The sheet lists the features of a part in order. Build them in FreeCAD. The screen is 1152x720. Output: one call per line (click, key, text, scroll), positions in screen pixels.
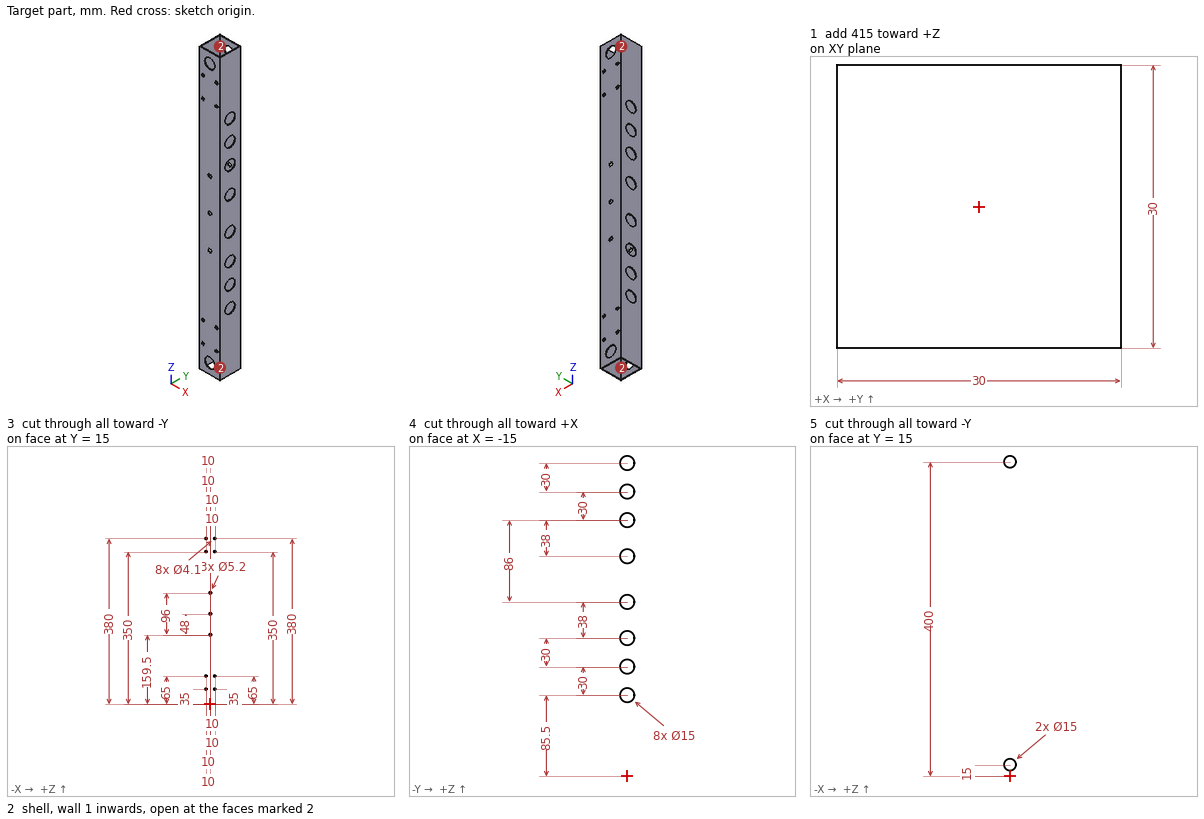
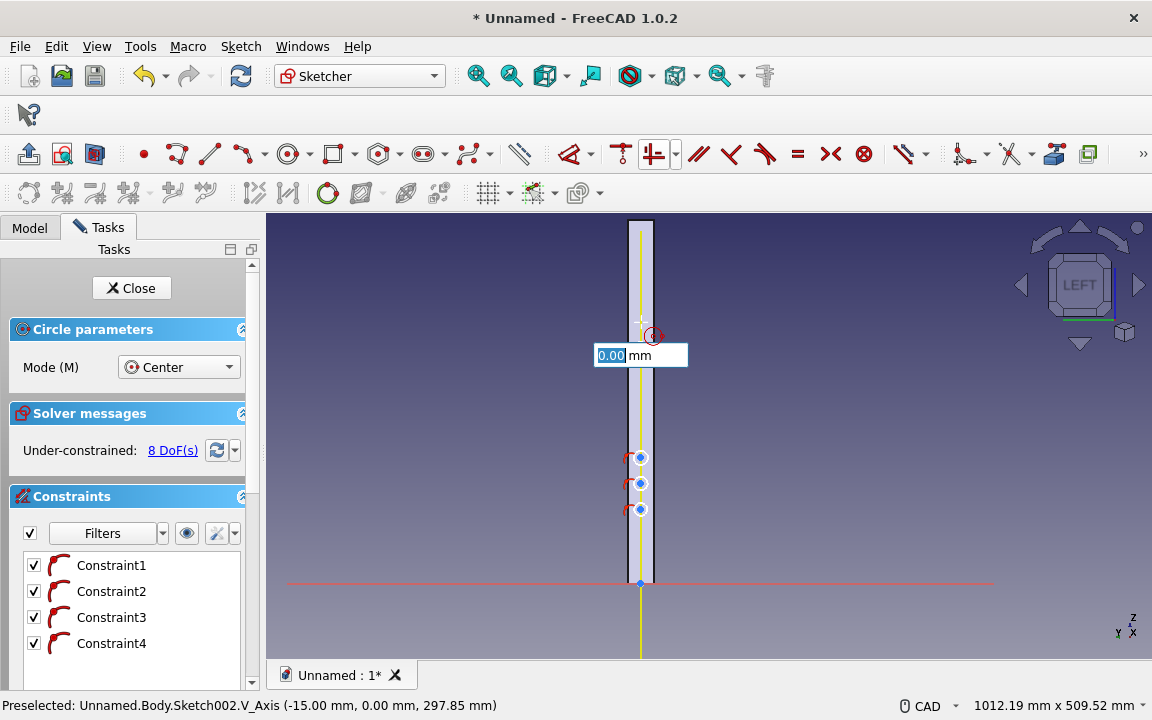
scroll(647, 319, up, 5)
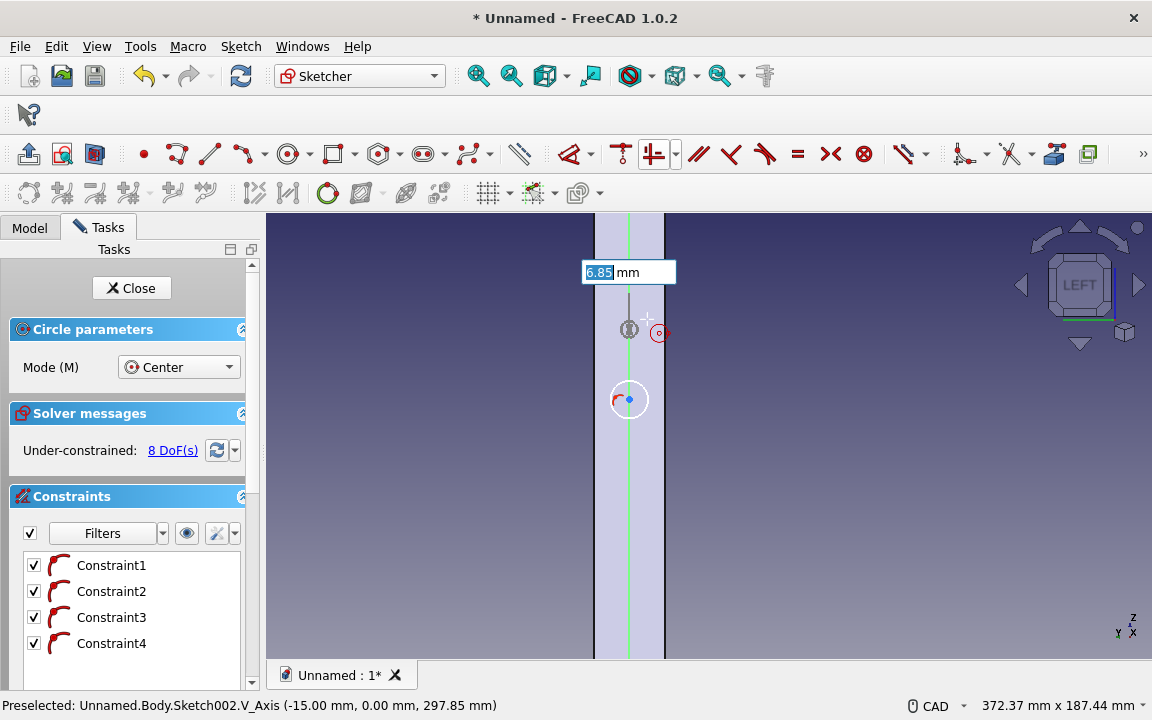
click(646, 319)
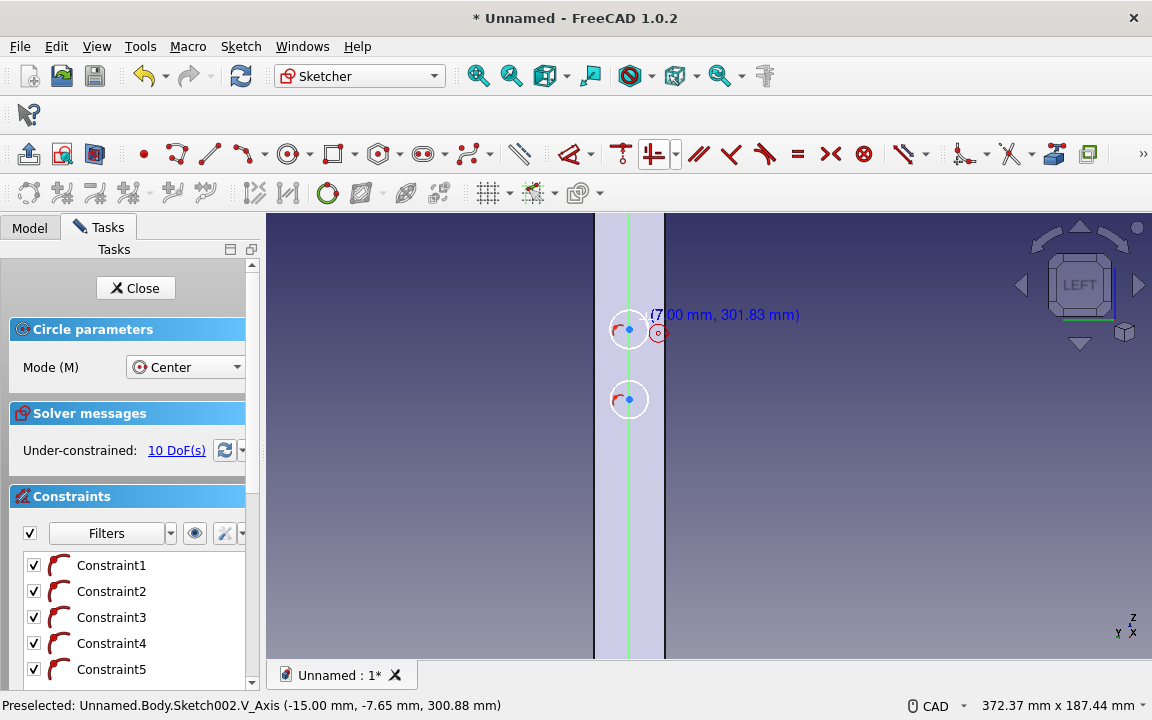
scroll(629, 254, up, 2)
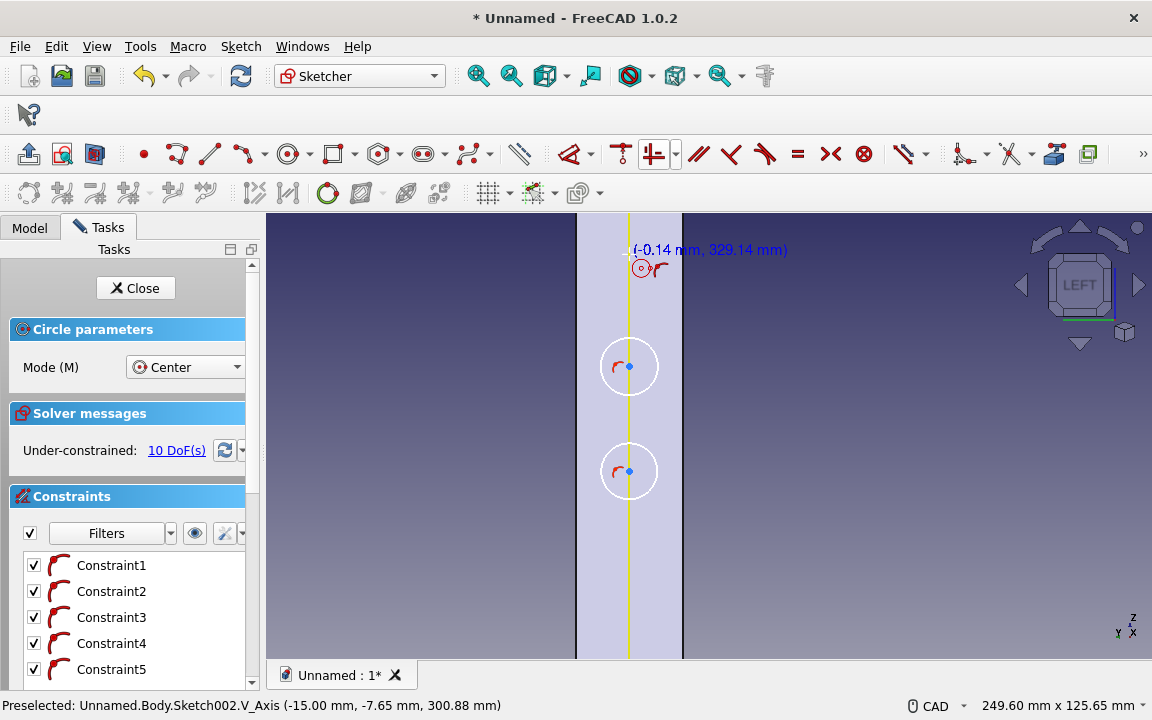
scroll(644, 308, down, 7)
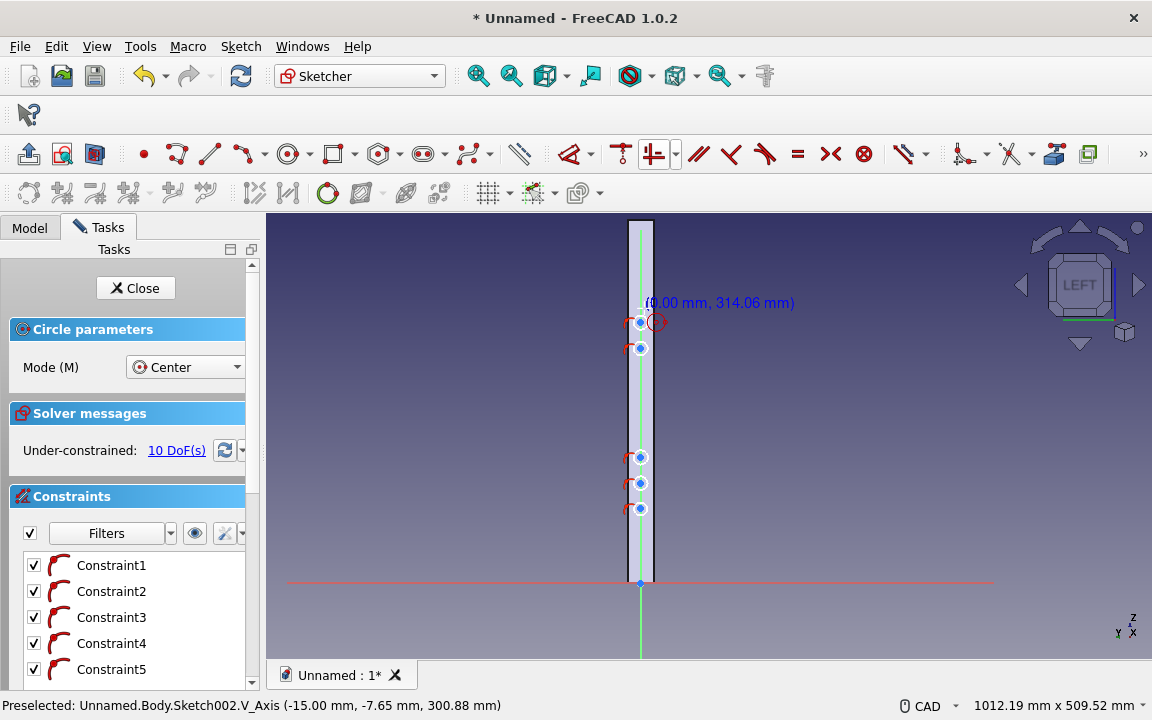
click(641, 295)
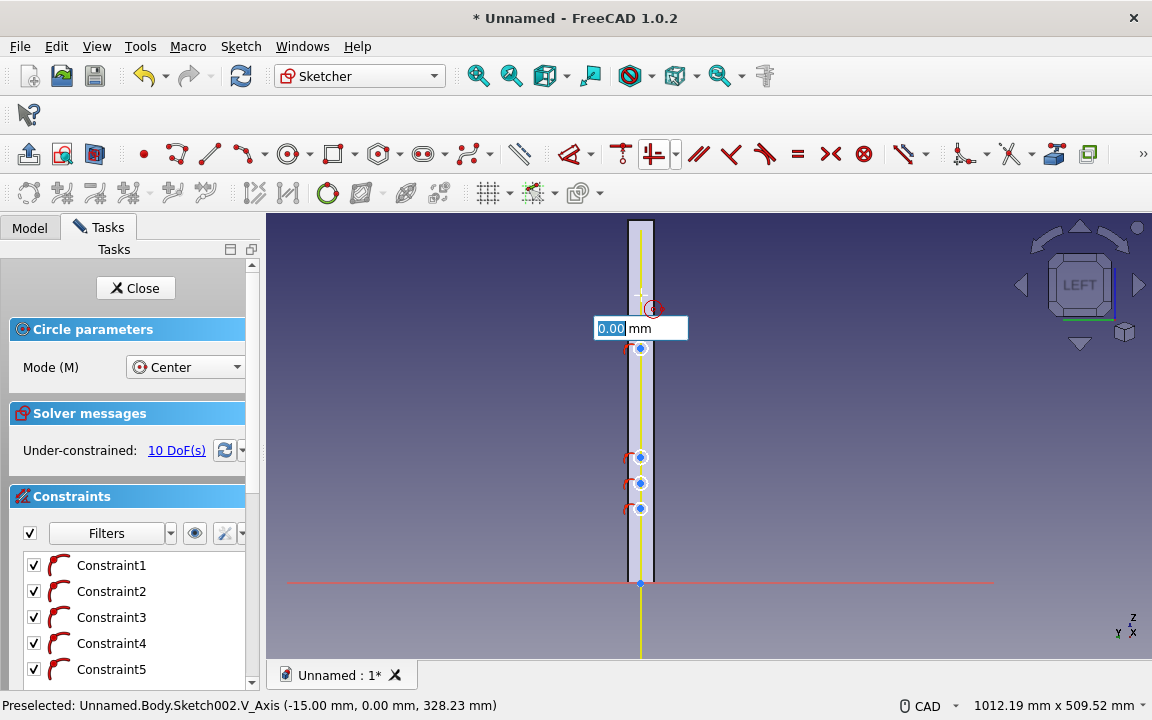
scroll(647, 293, up, 5)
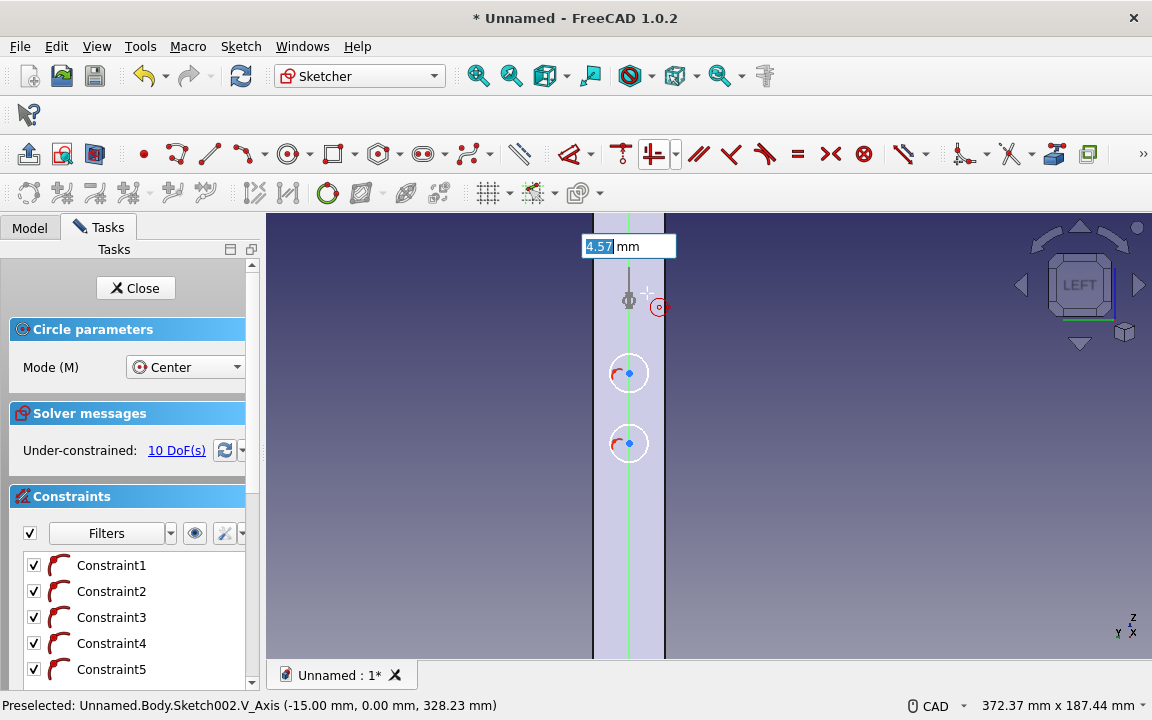
click(646, 292)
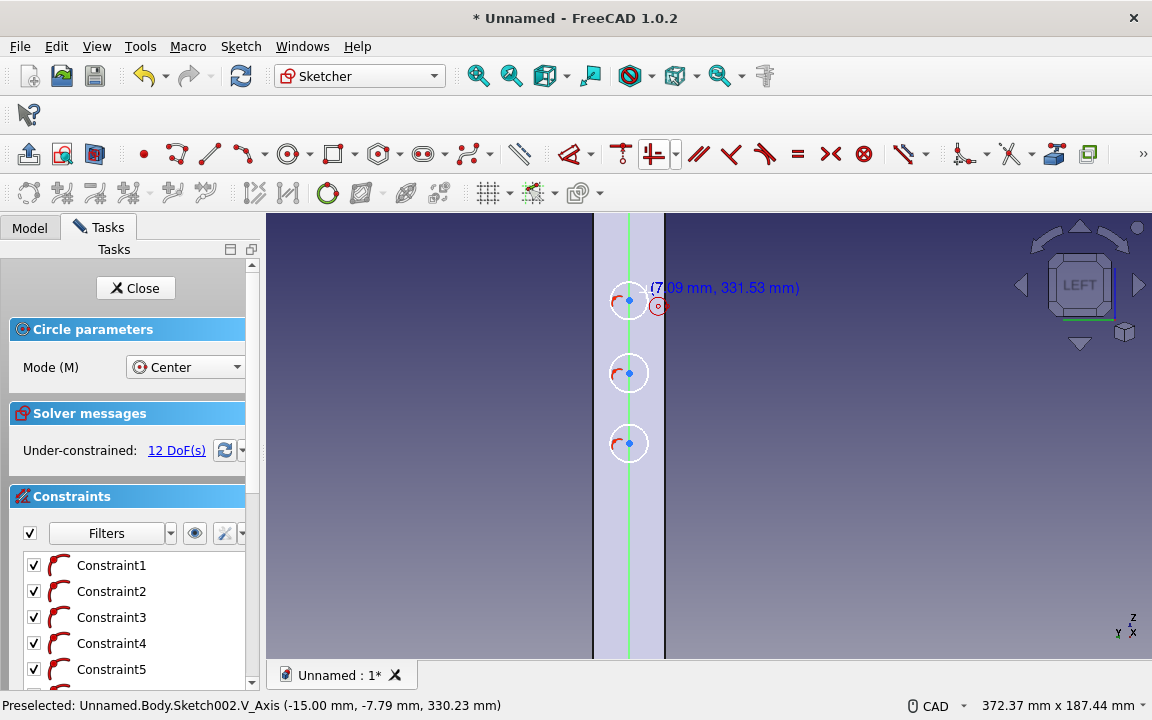
scroll(647, 293, down, 5)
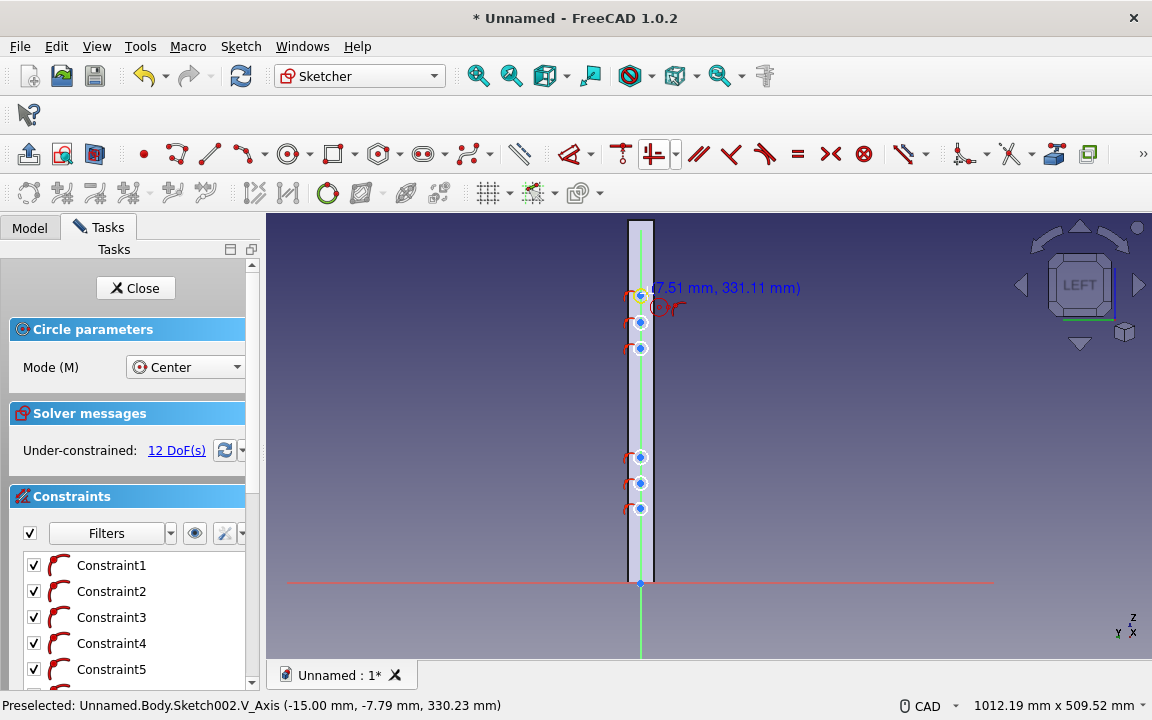
scroll(641, 423, up, 7)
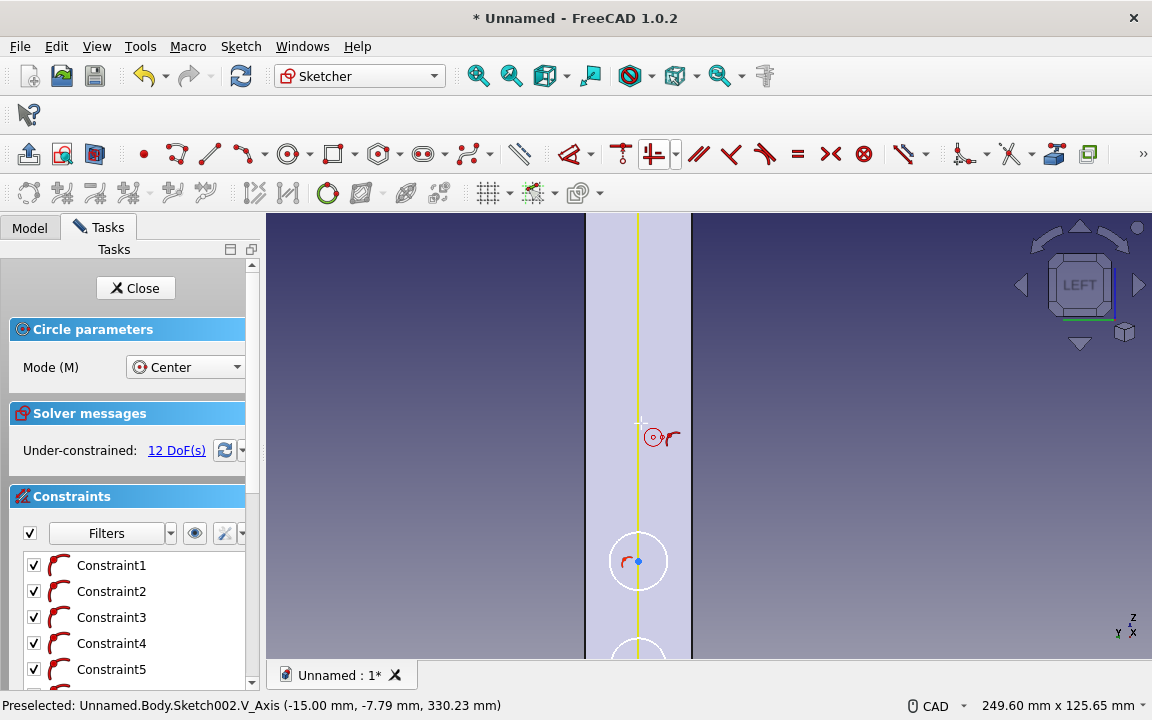
scroll(641, 424, down, 7)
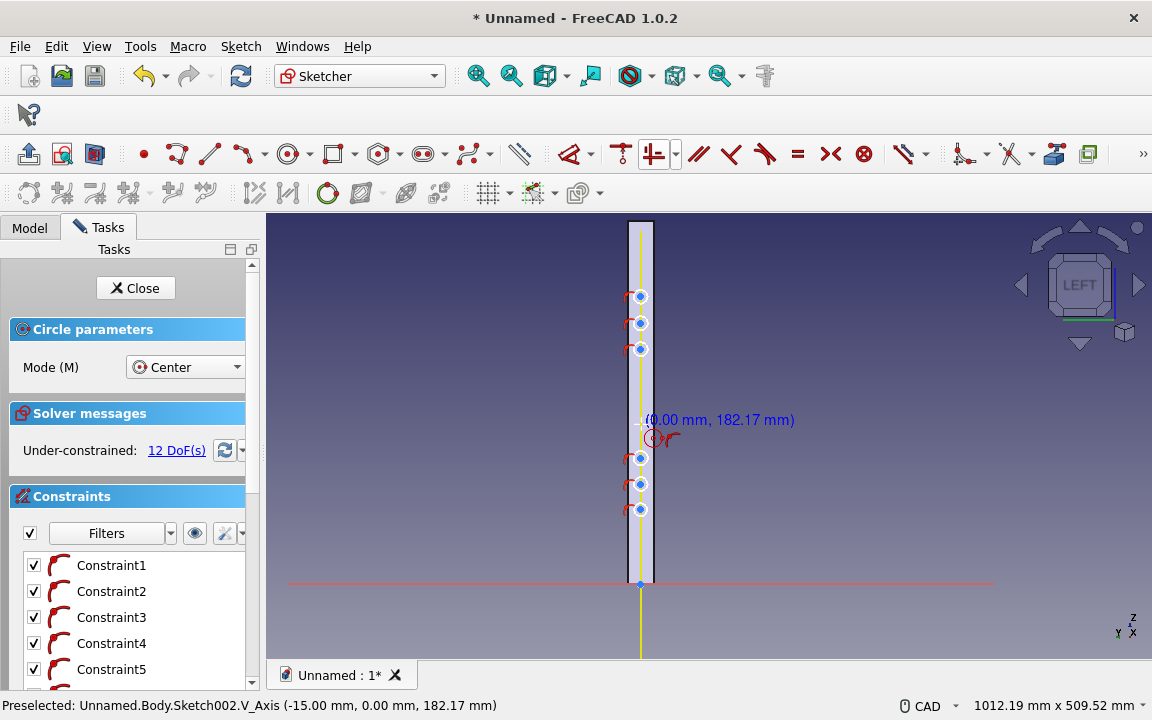
click(641, 423)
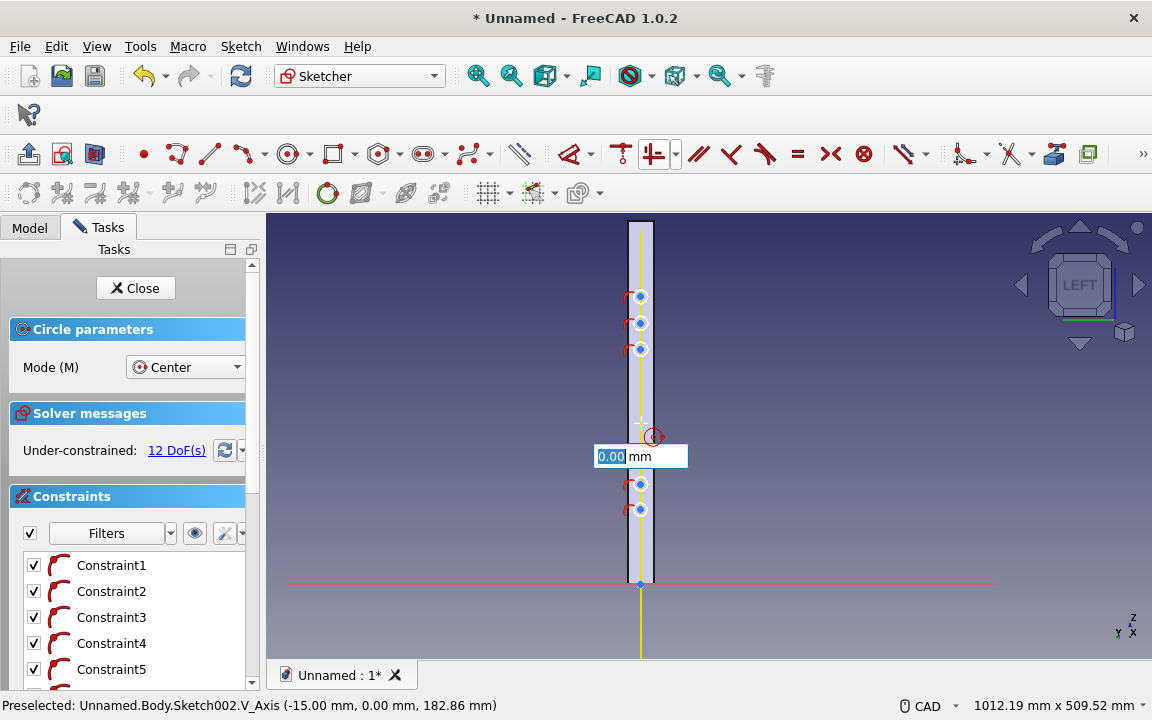
scroll(647, 421, up, 5)